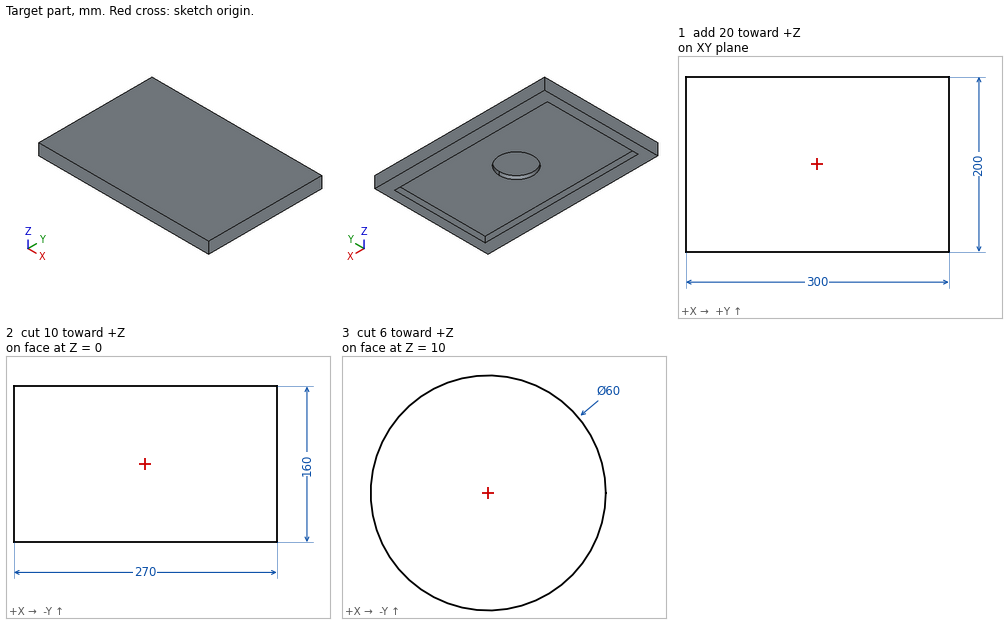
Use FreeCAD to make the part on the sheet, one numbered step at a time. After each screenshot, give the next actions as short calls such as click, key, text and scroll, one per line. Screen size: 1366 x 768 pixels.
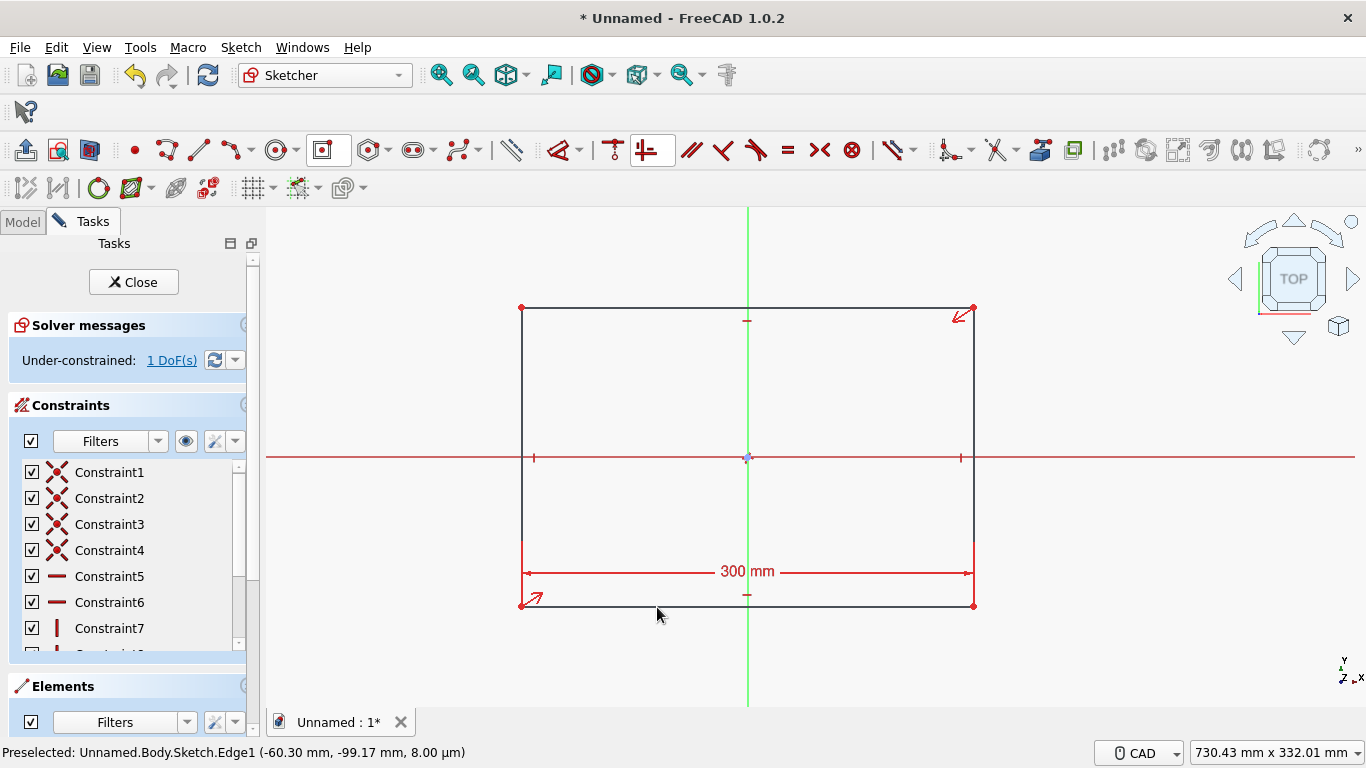
click(974, 517)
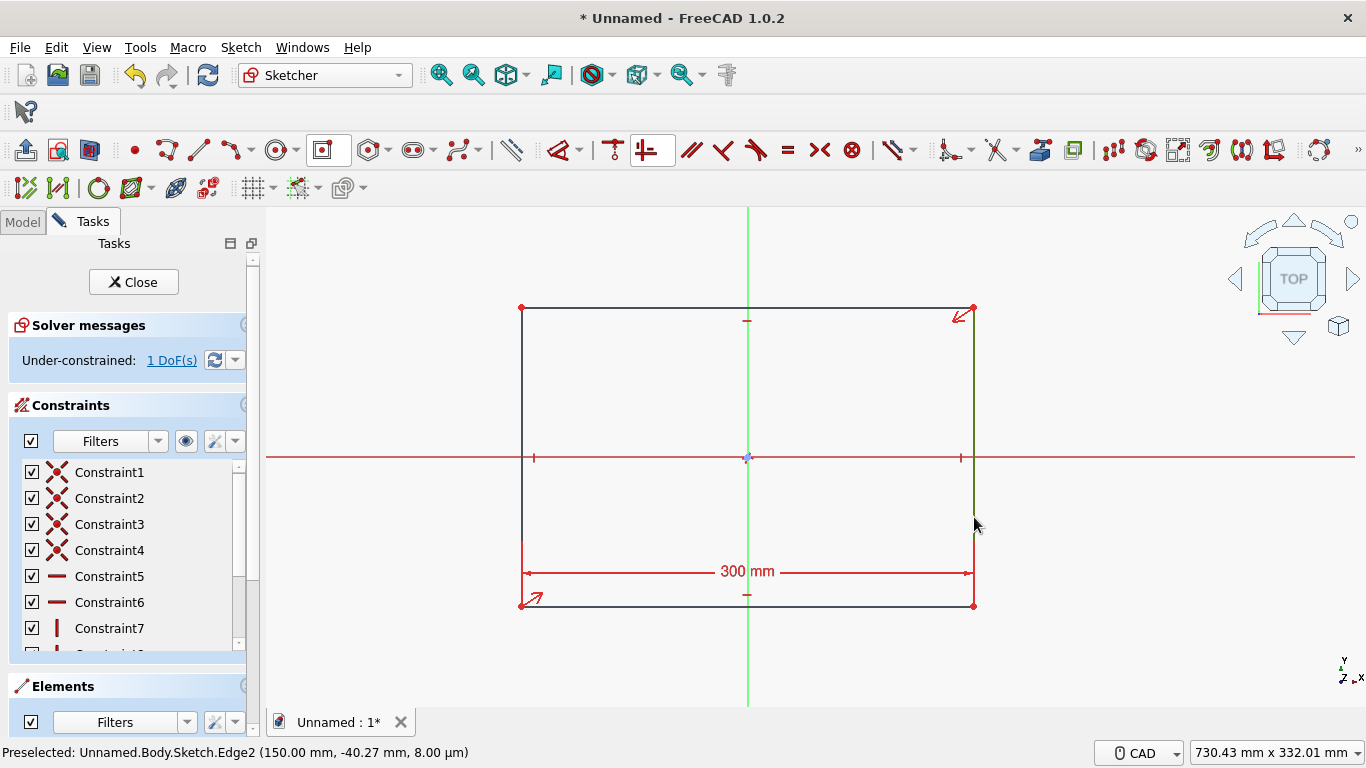
key(i)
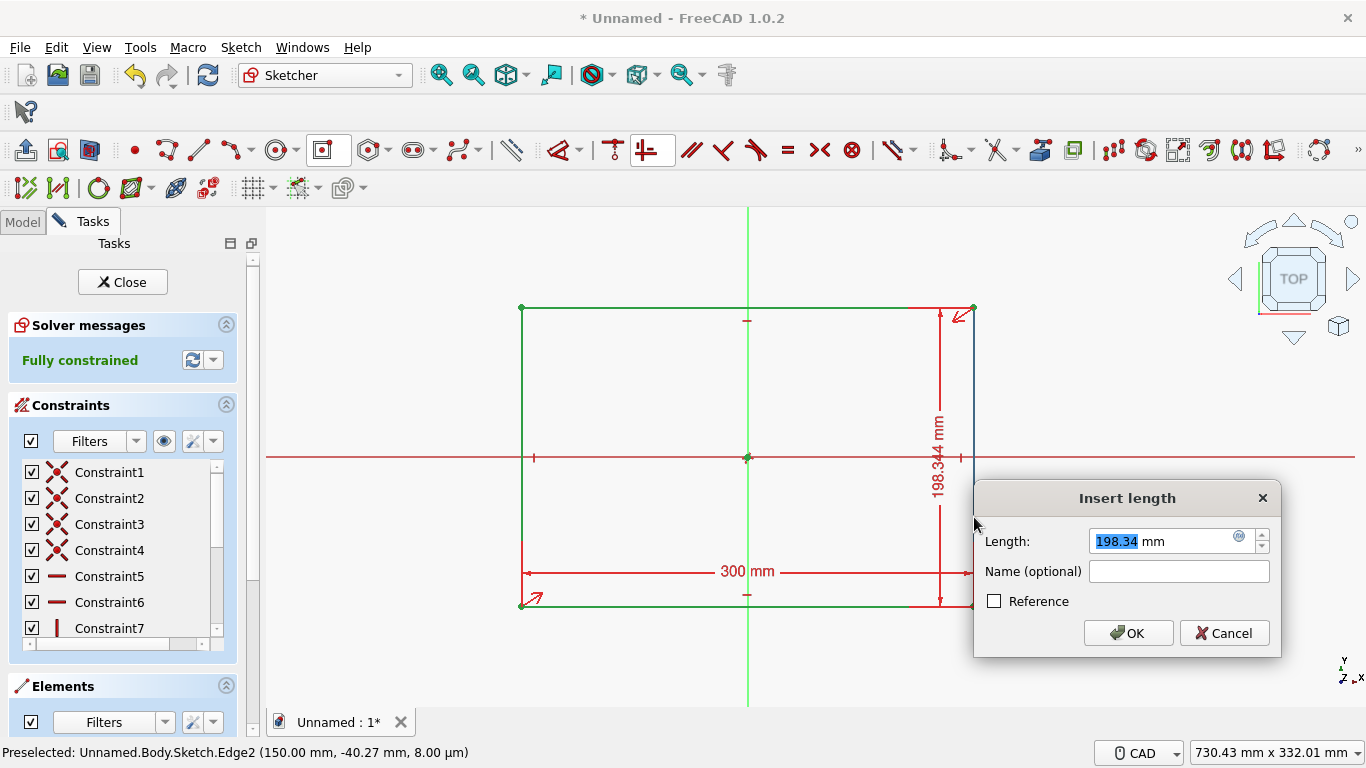
text(200)
key(Return)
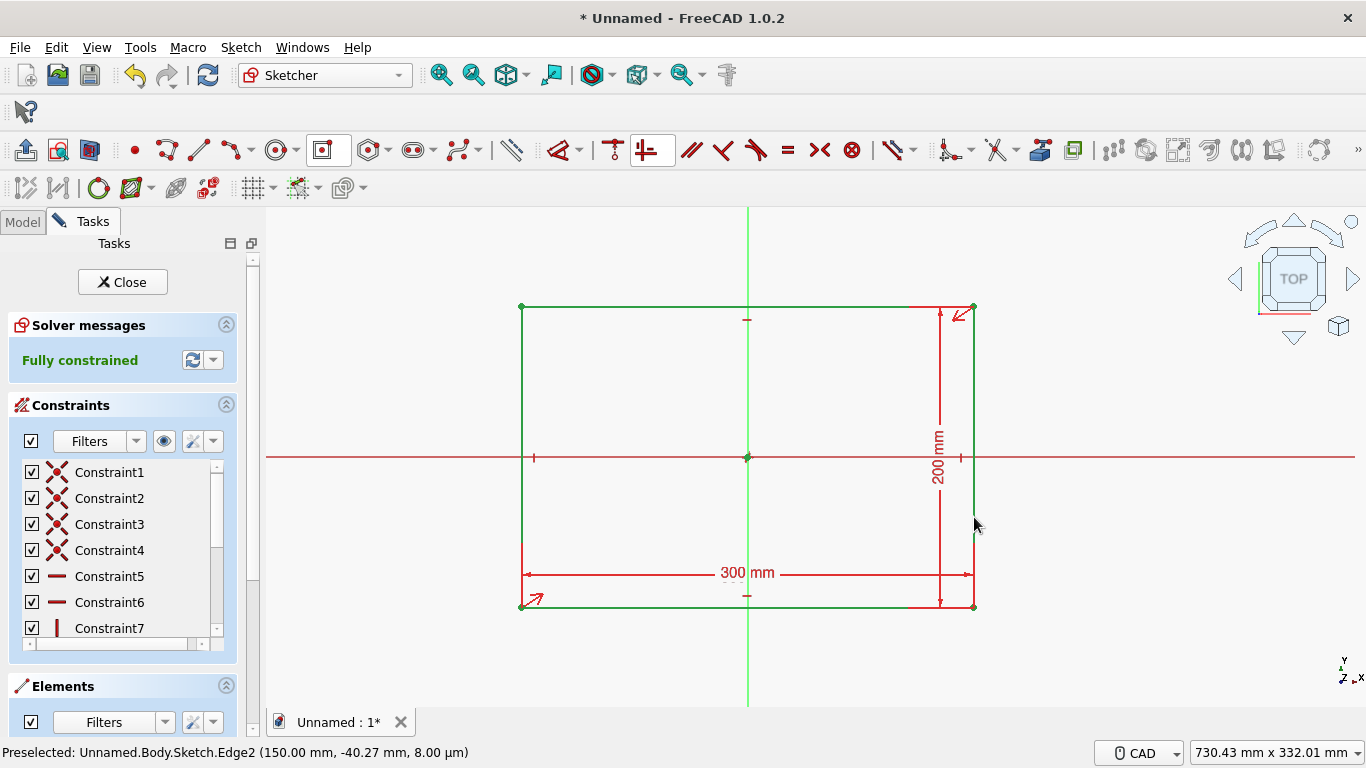
click(123, 282)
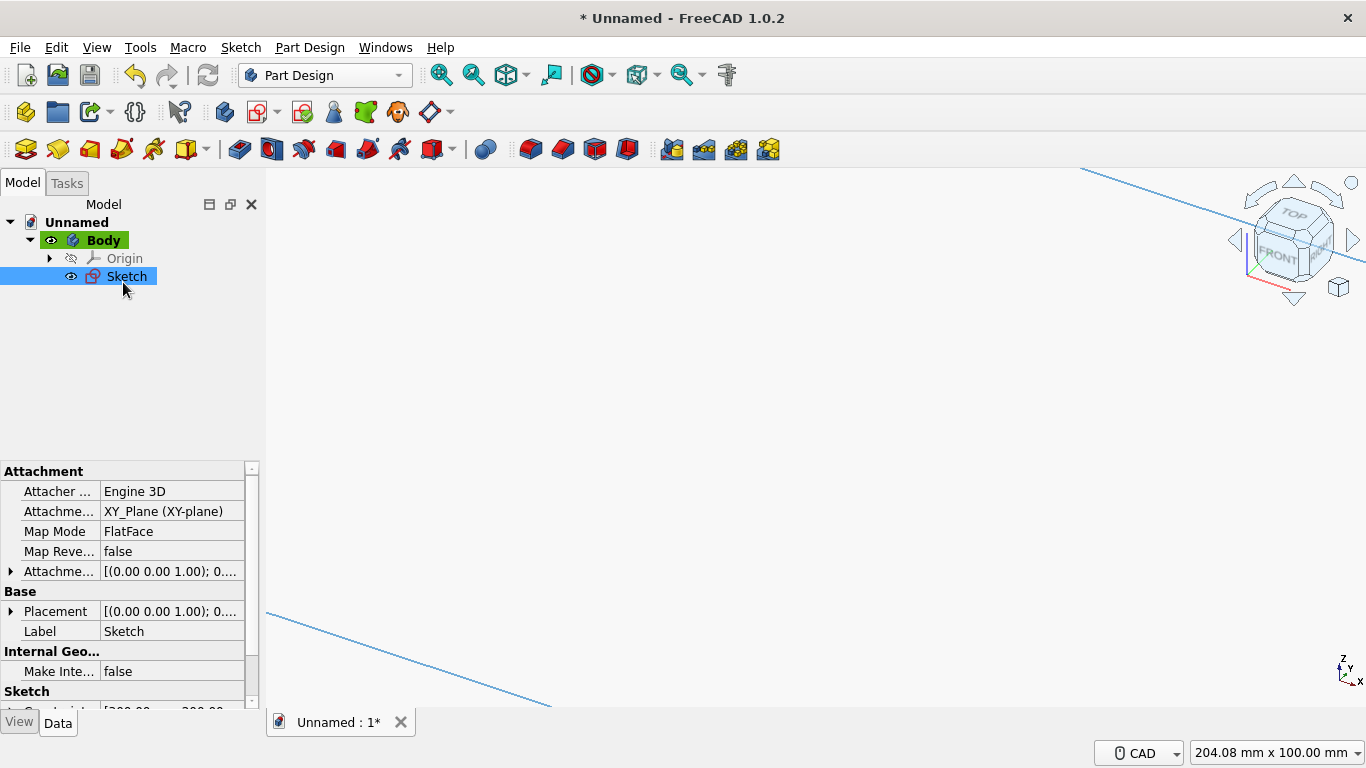
click(26, 150)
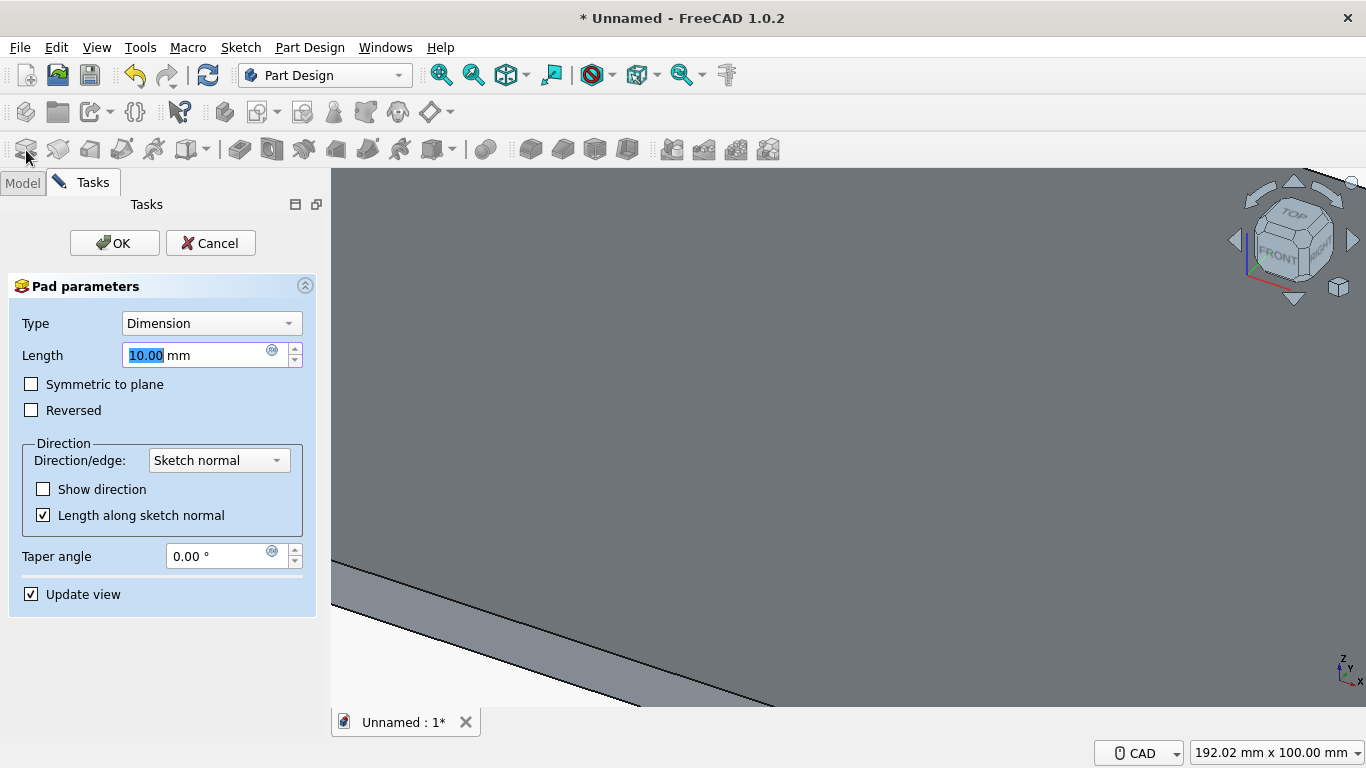
text(20)
key(Tab)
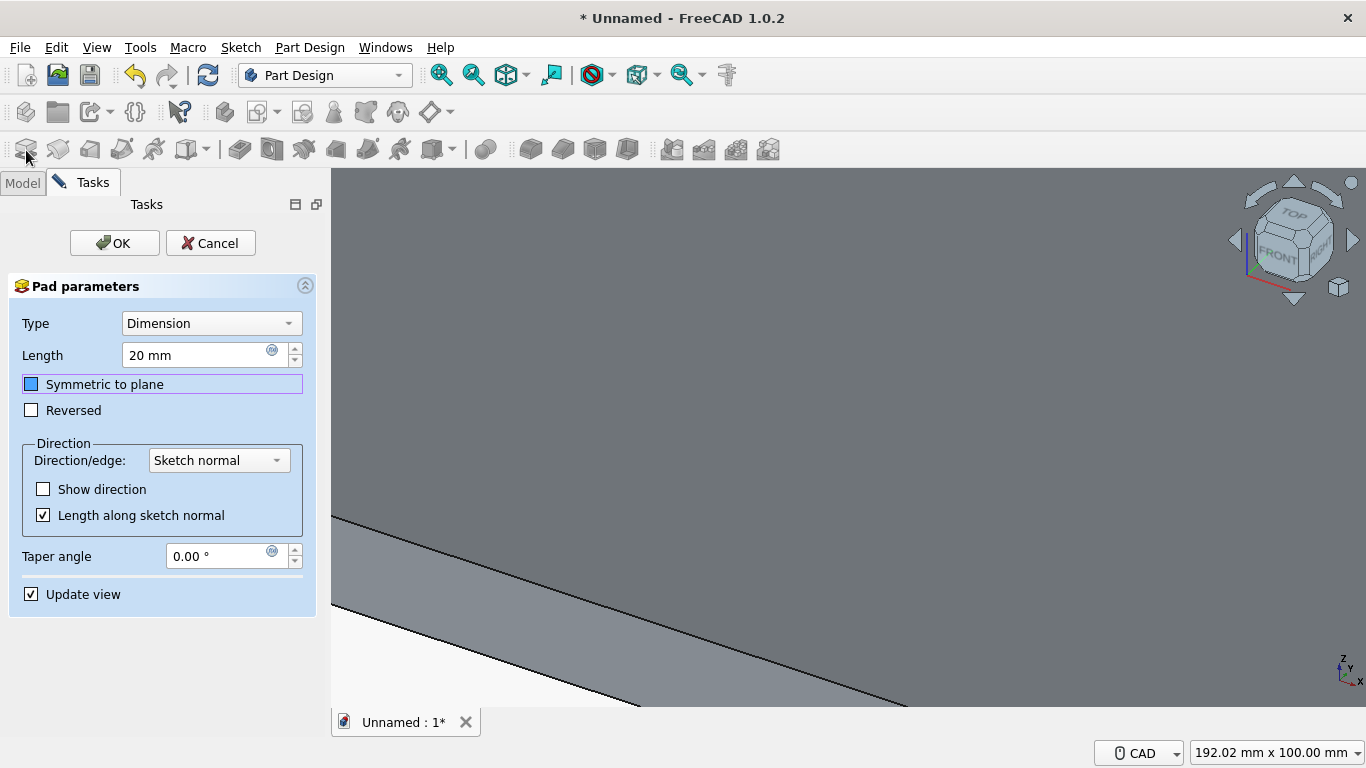
click(115, 243)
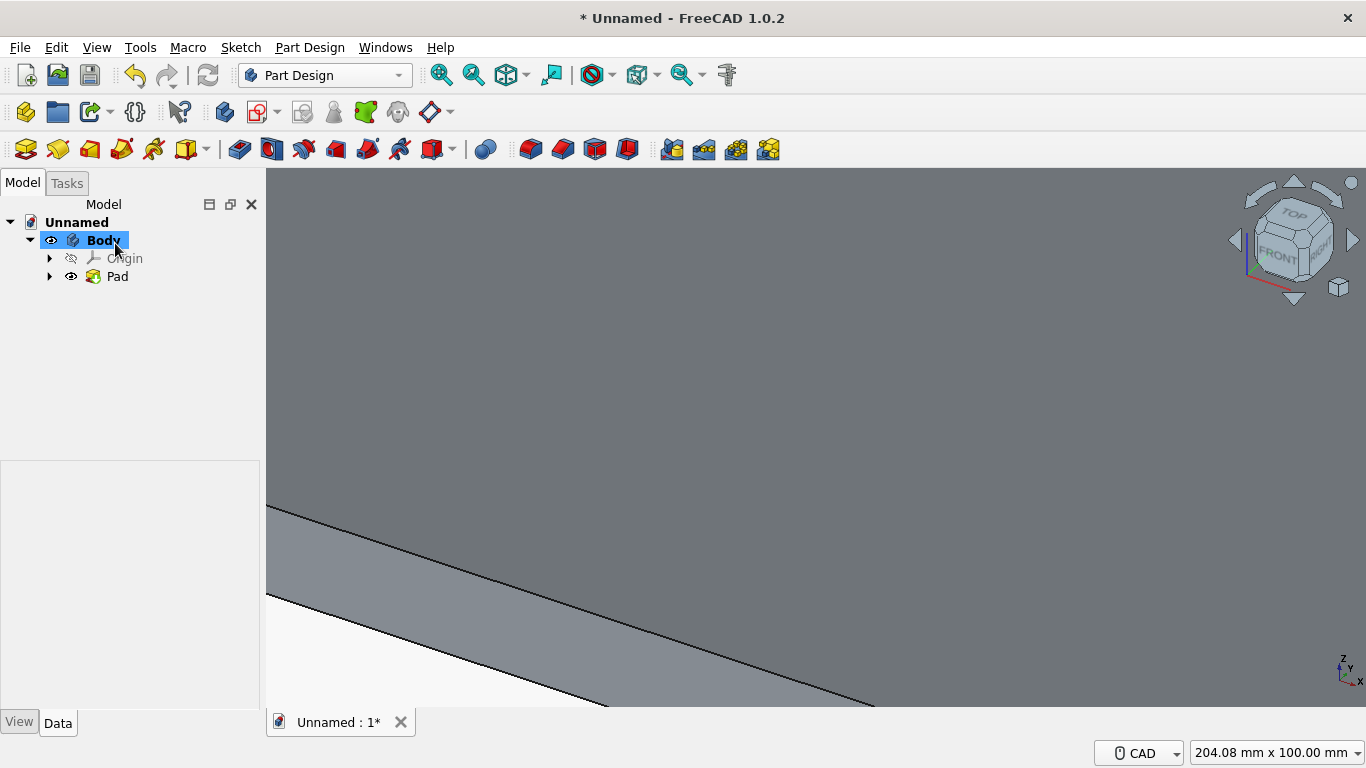
key(v)
key(f)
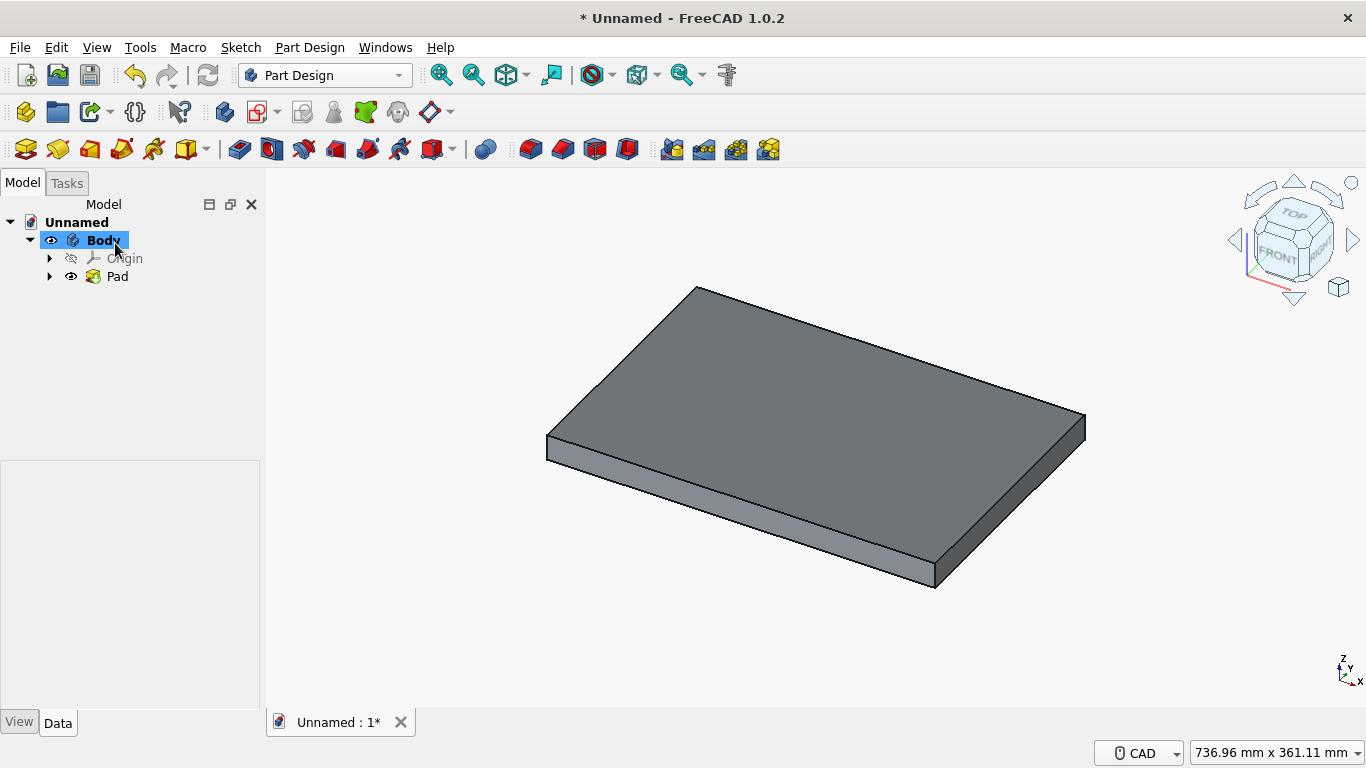
key(5)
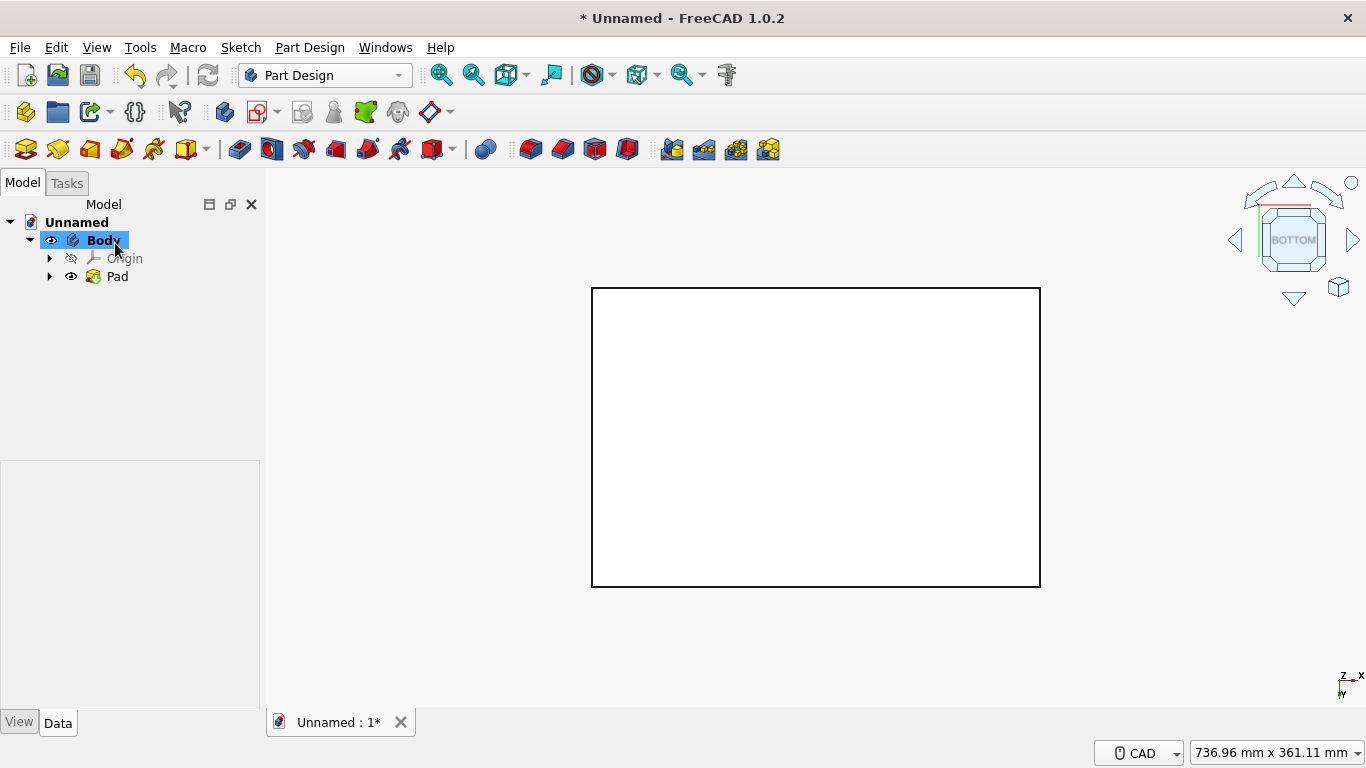
click(880, 436)